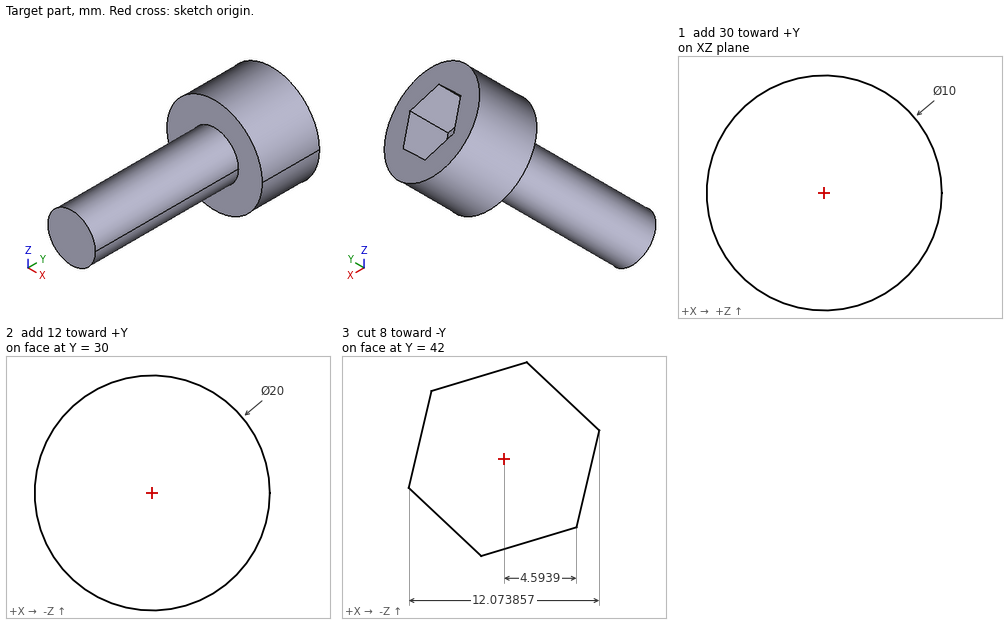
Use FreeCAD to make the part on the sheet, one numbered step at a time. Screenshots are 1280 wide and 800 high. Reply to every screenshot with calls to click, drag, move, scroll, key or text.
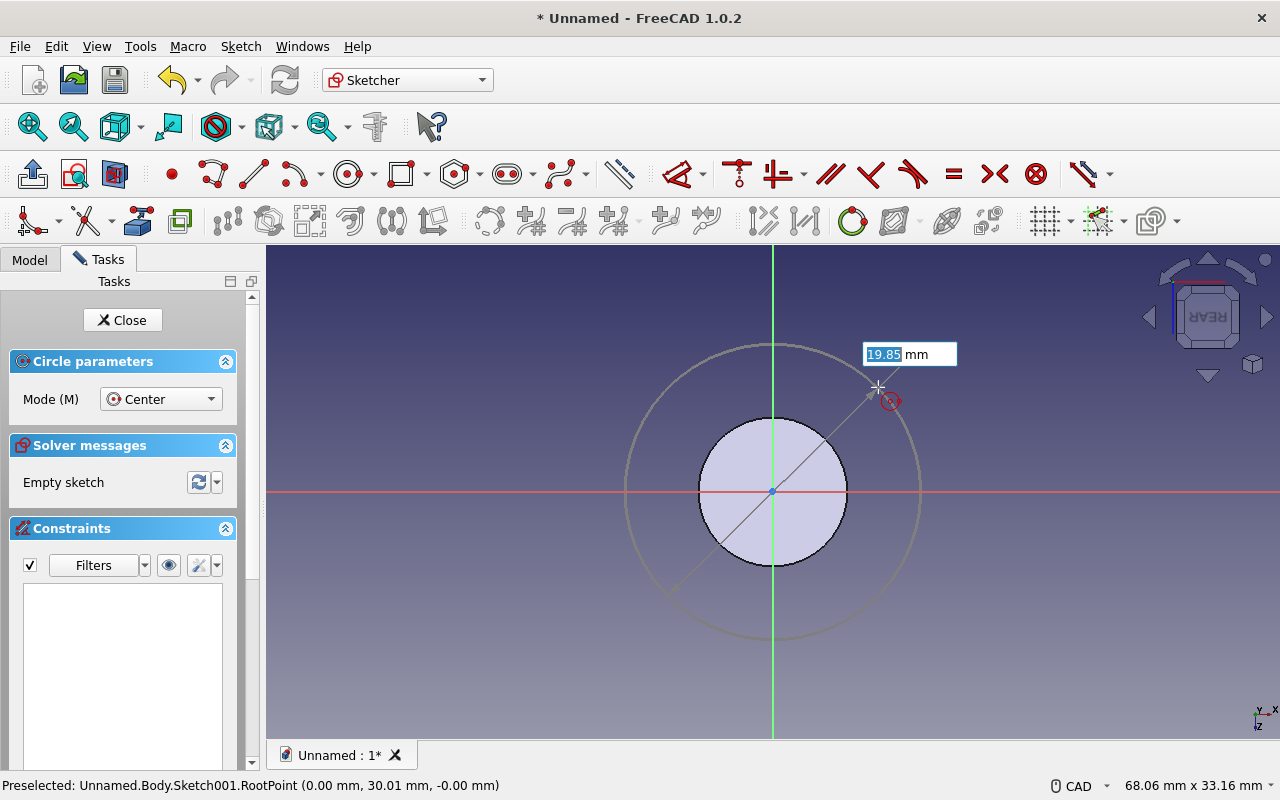
text(20)
key(Return)
key(Escape)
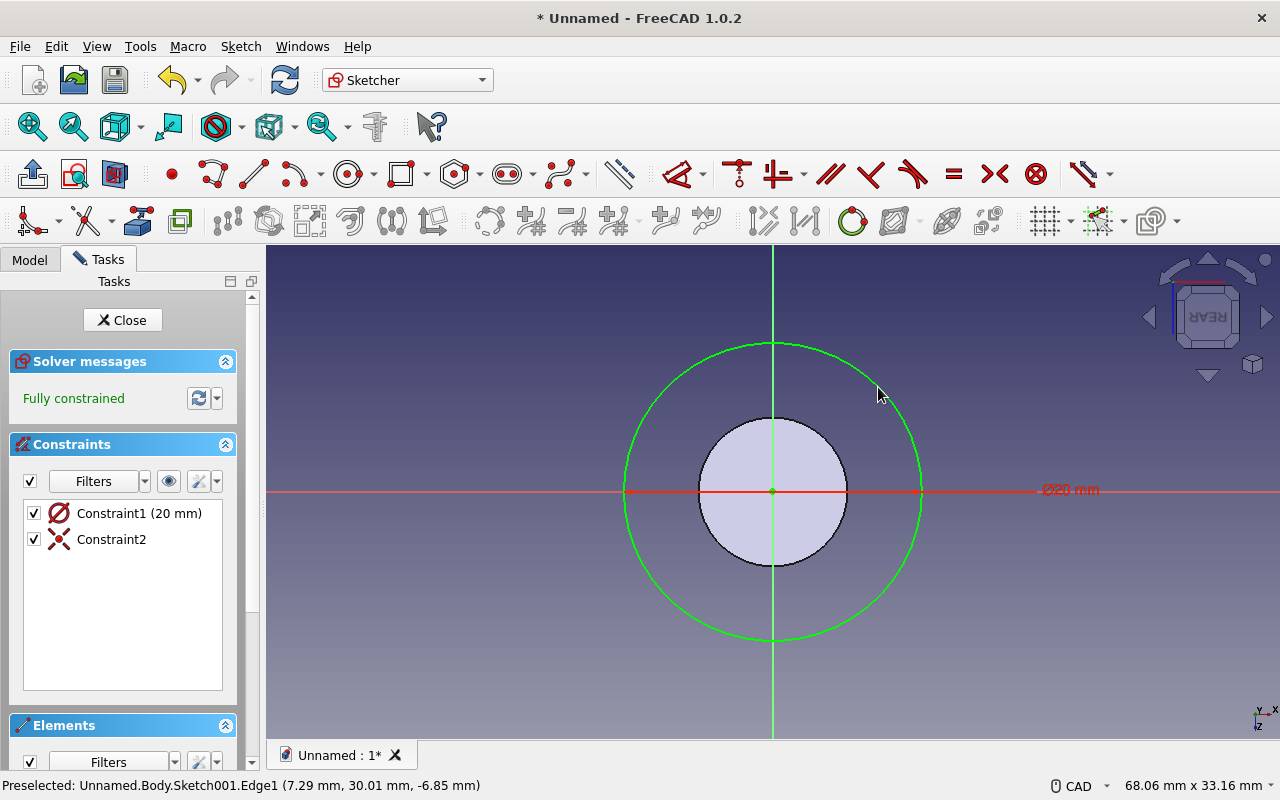
click(123, 320)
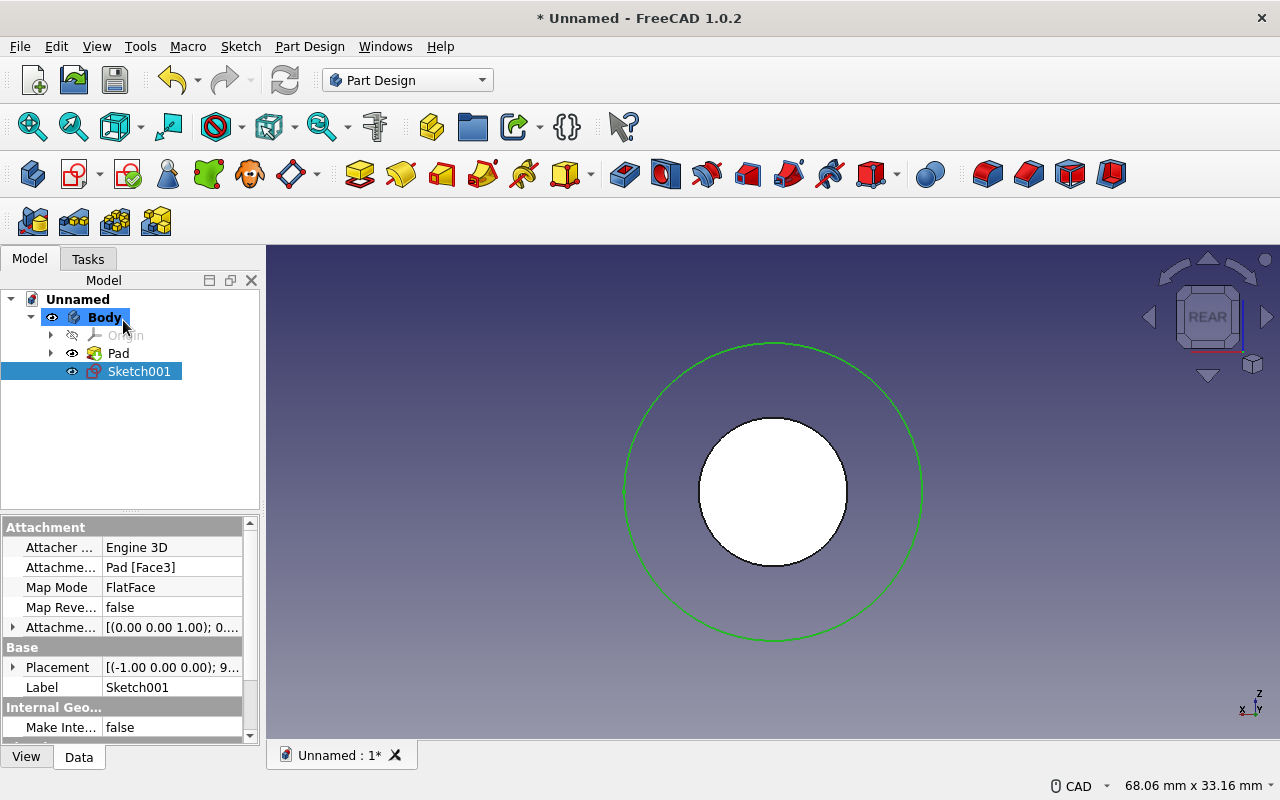
click(360, 174)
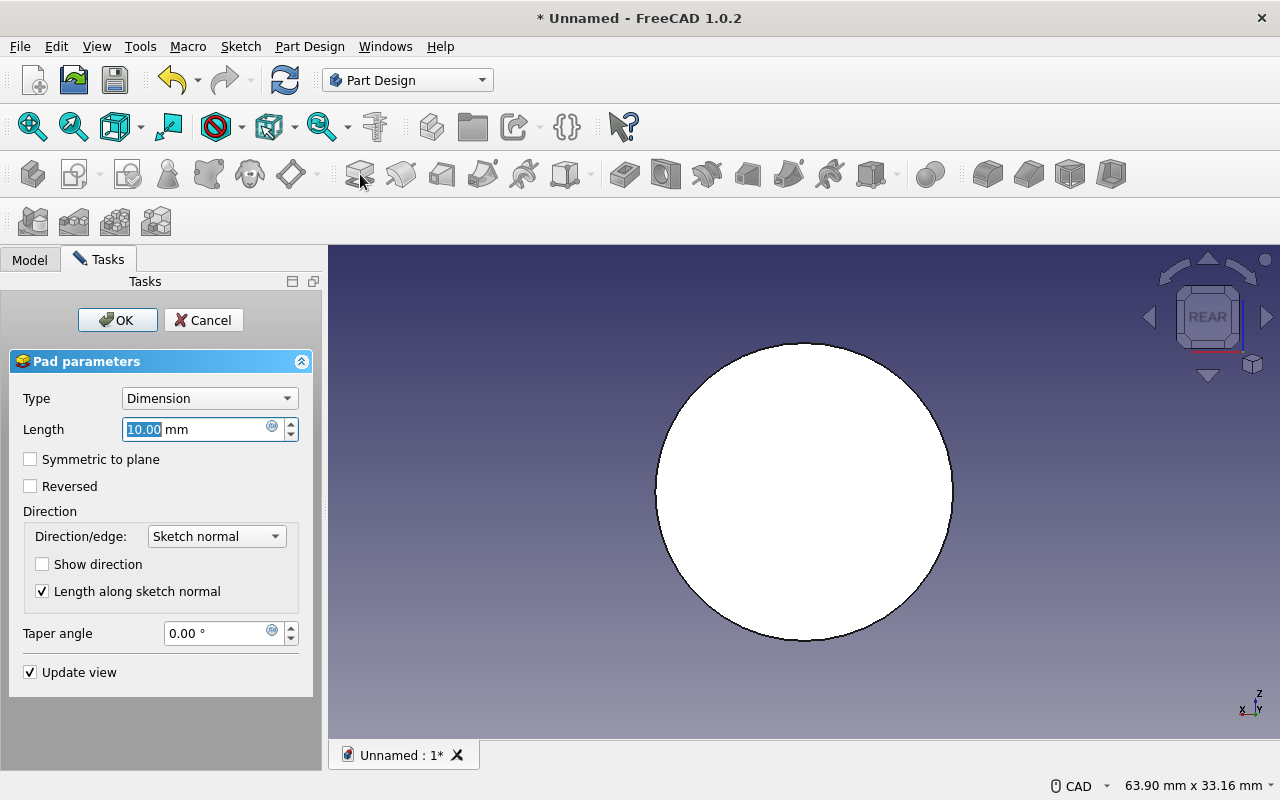
text(12)
key(Tab)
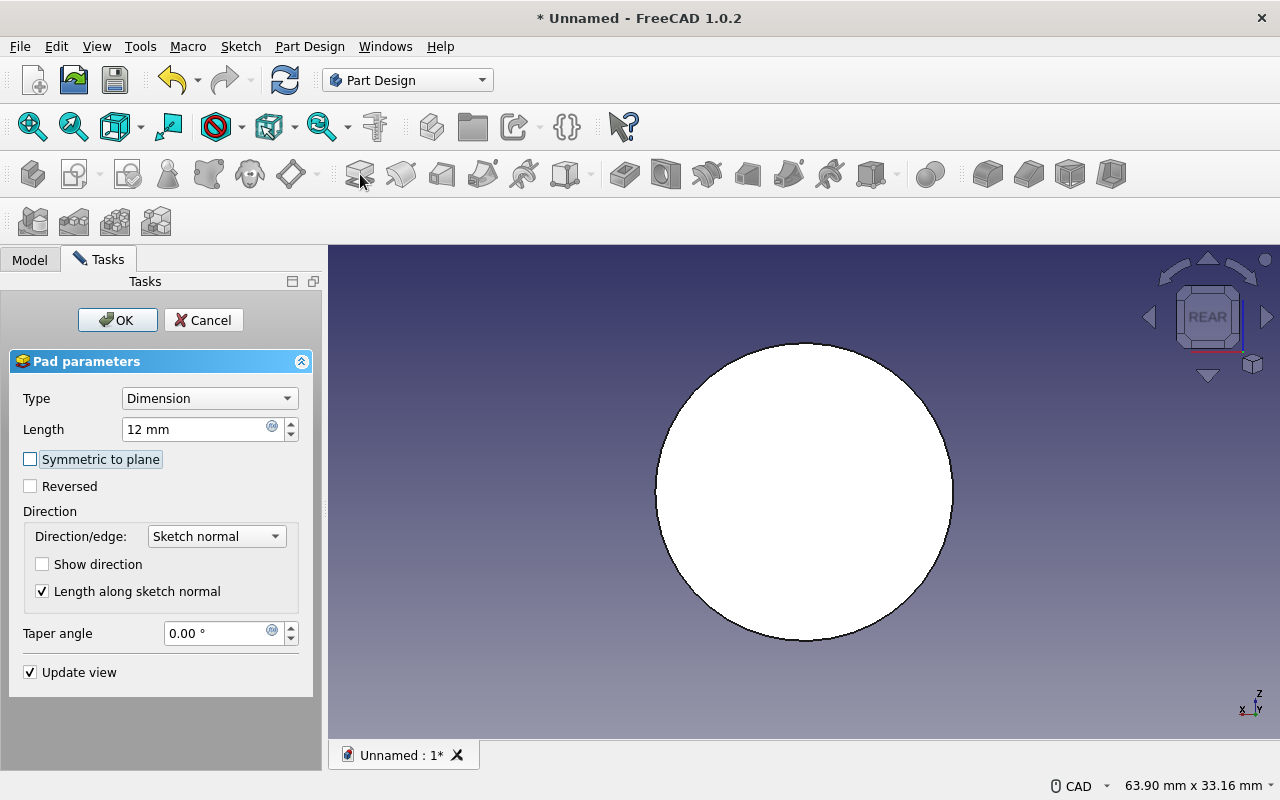
click(118, 320)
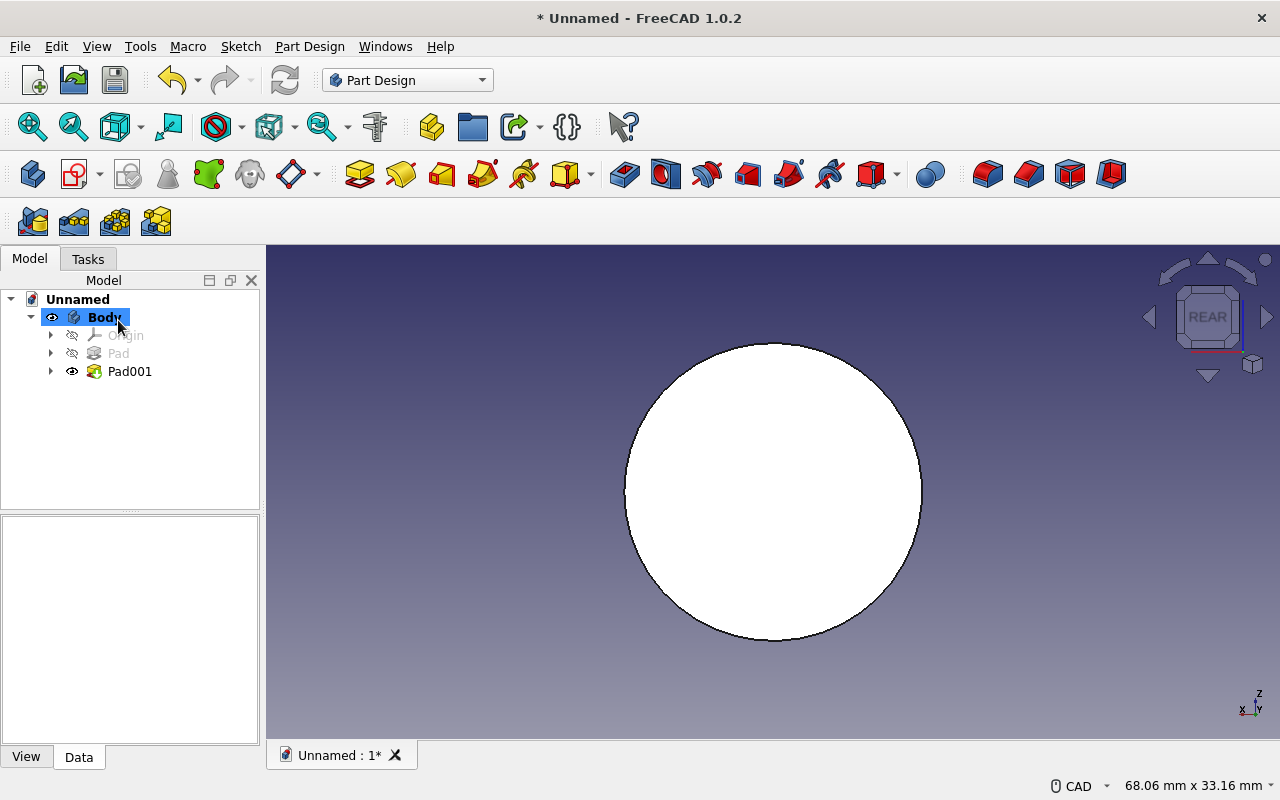
click(773, 491)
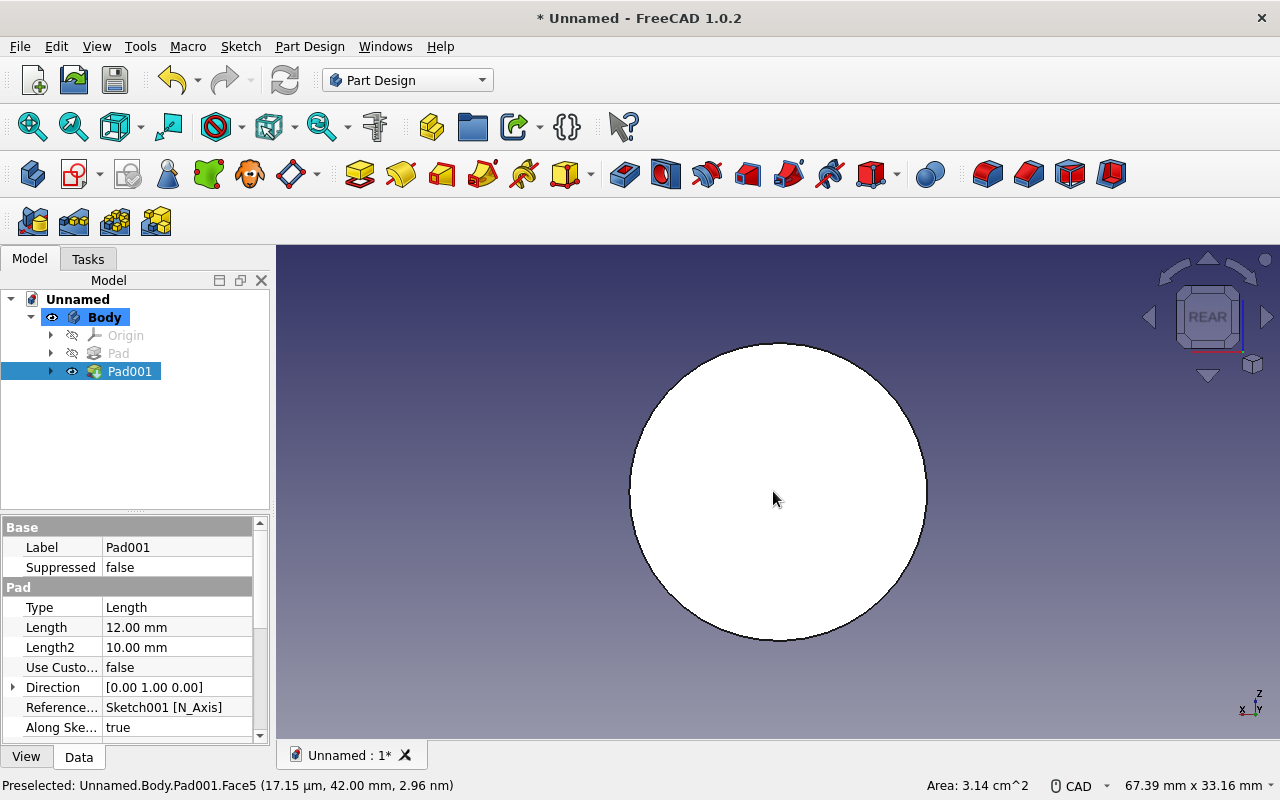
click(74, 174)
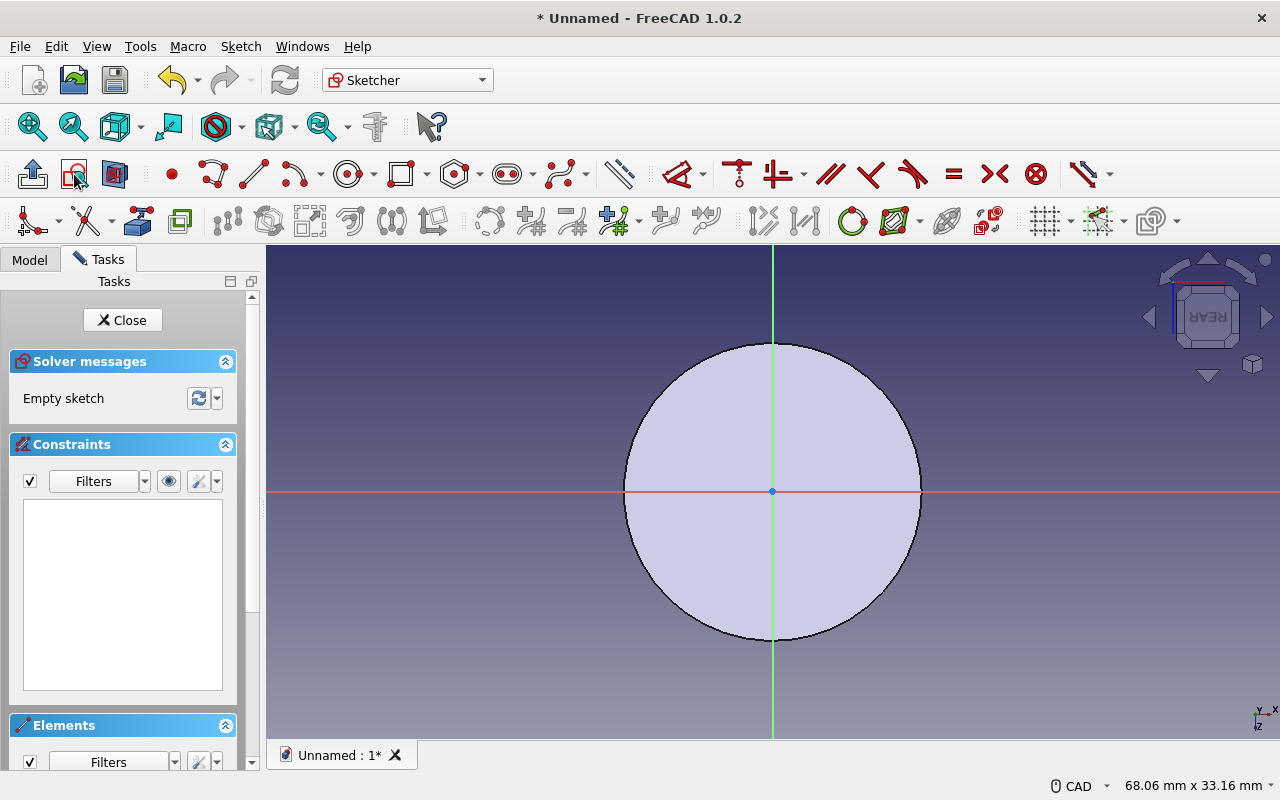
scroll(856, 492, up, 3)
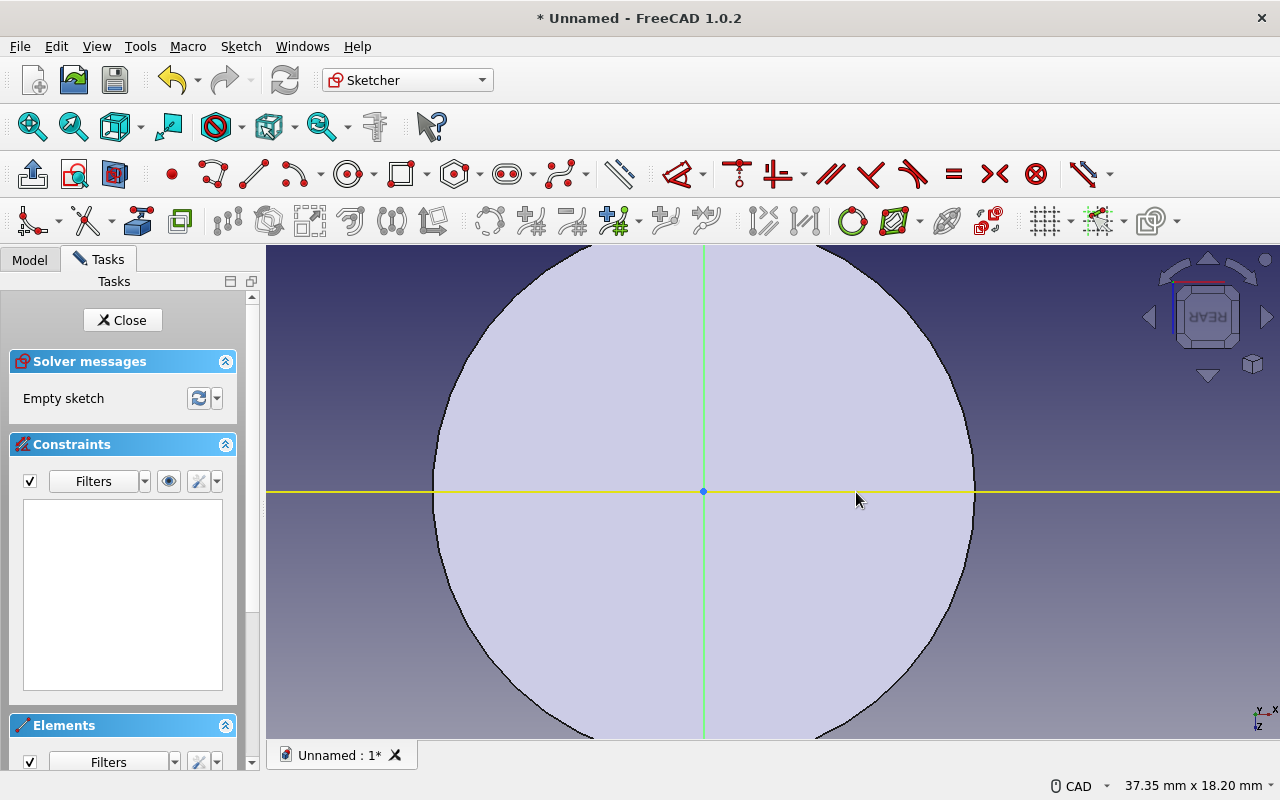
key(g)
key(p)
key(6)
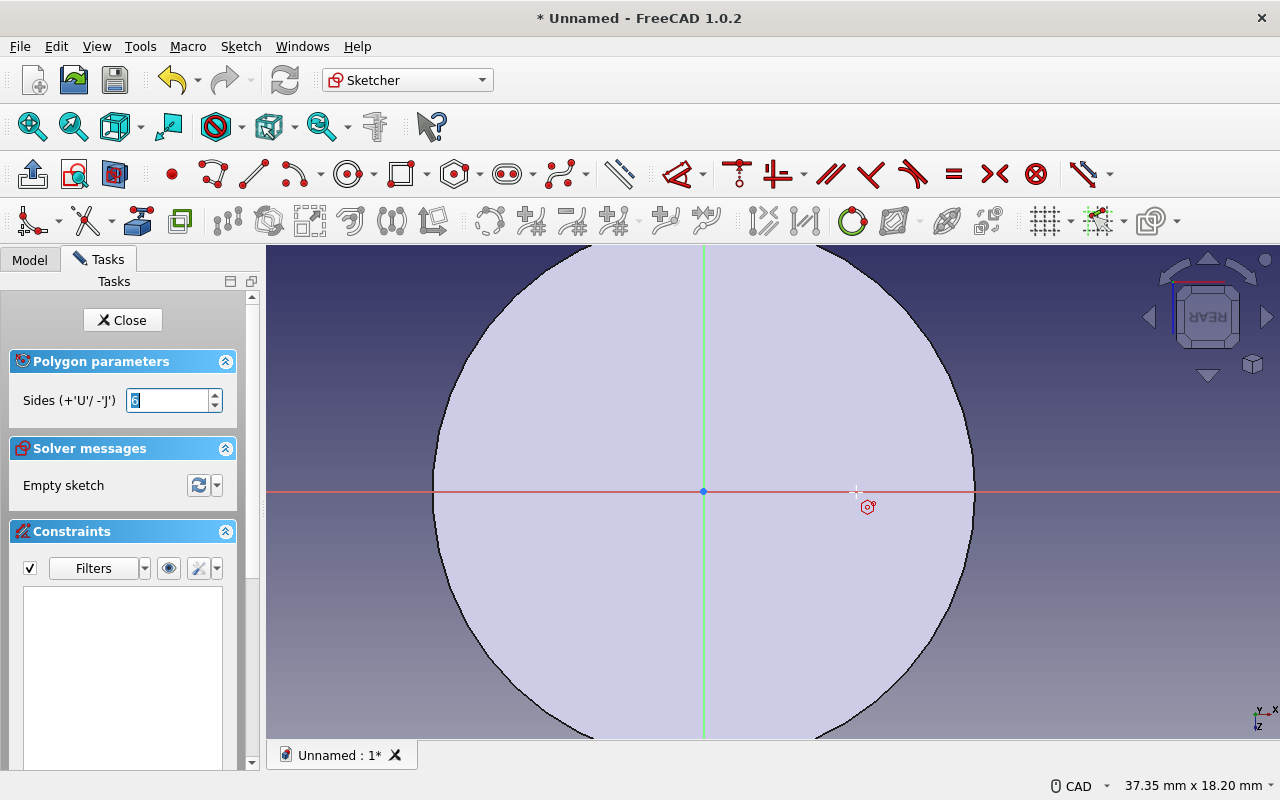
click(704, 492)